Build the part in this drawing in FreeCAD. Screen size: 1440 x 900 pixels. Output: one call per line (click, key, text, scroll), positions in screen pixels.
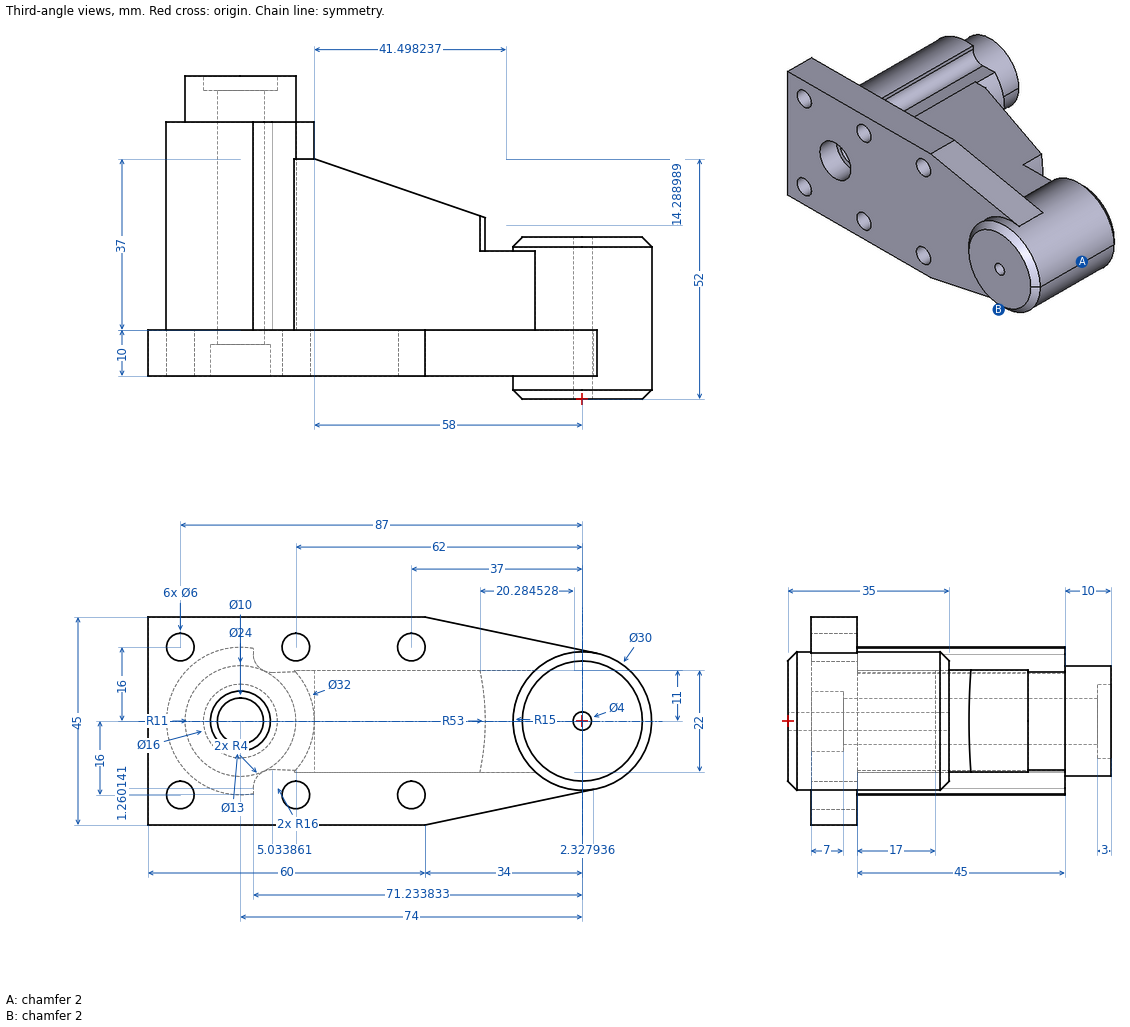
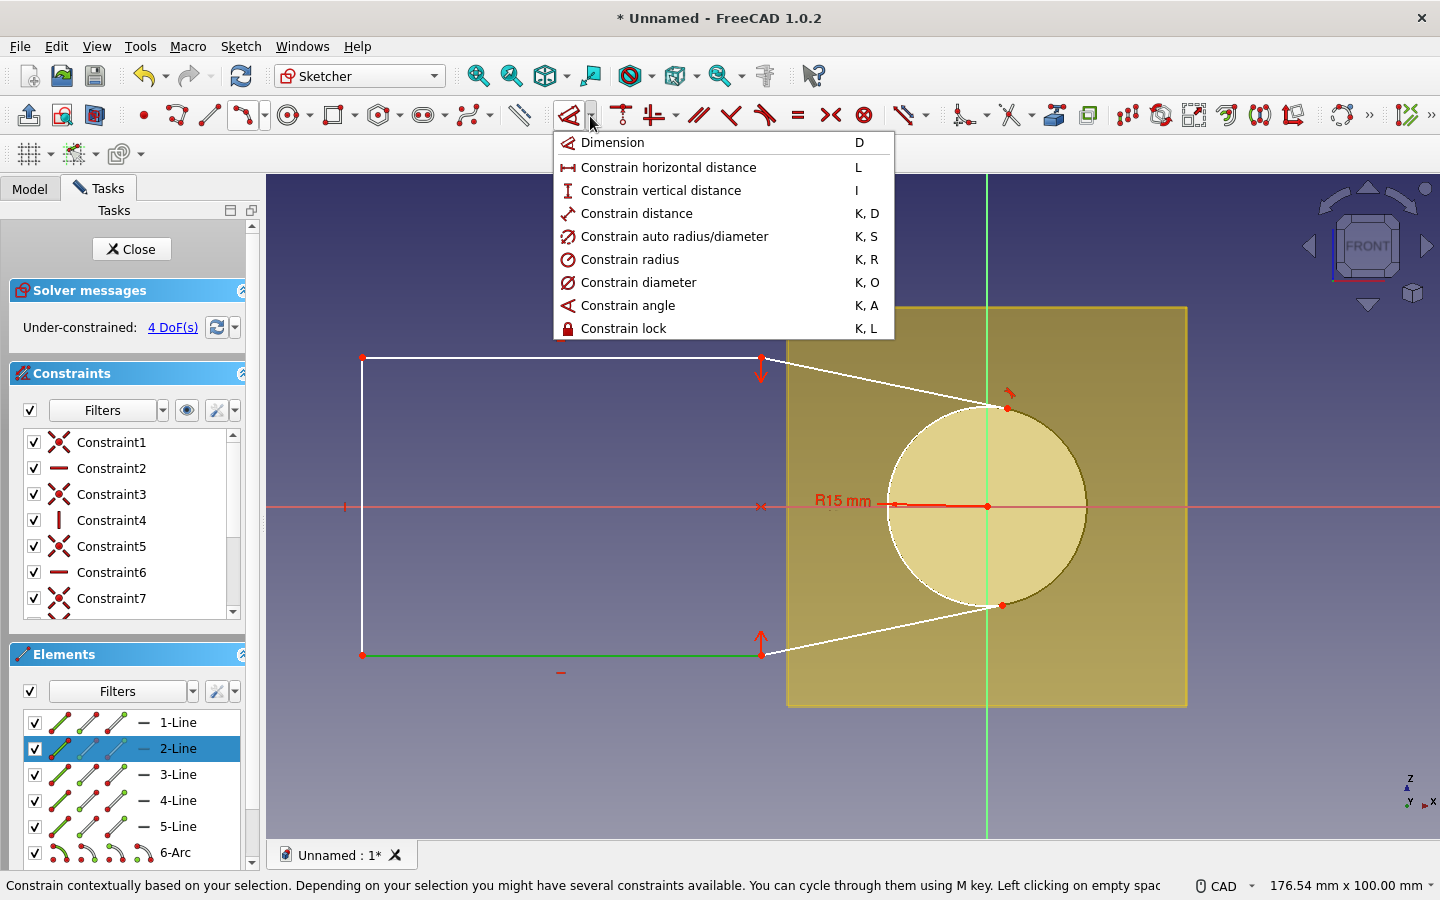
click(724, 168)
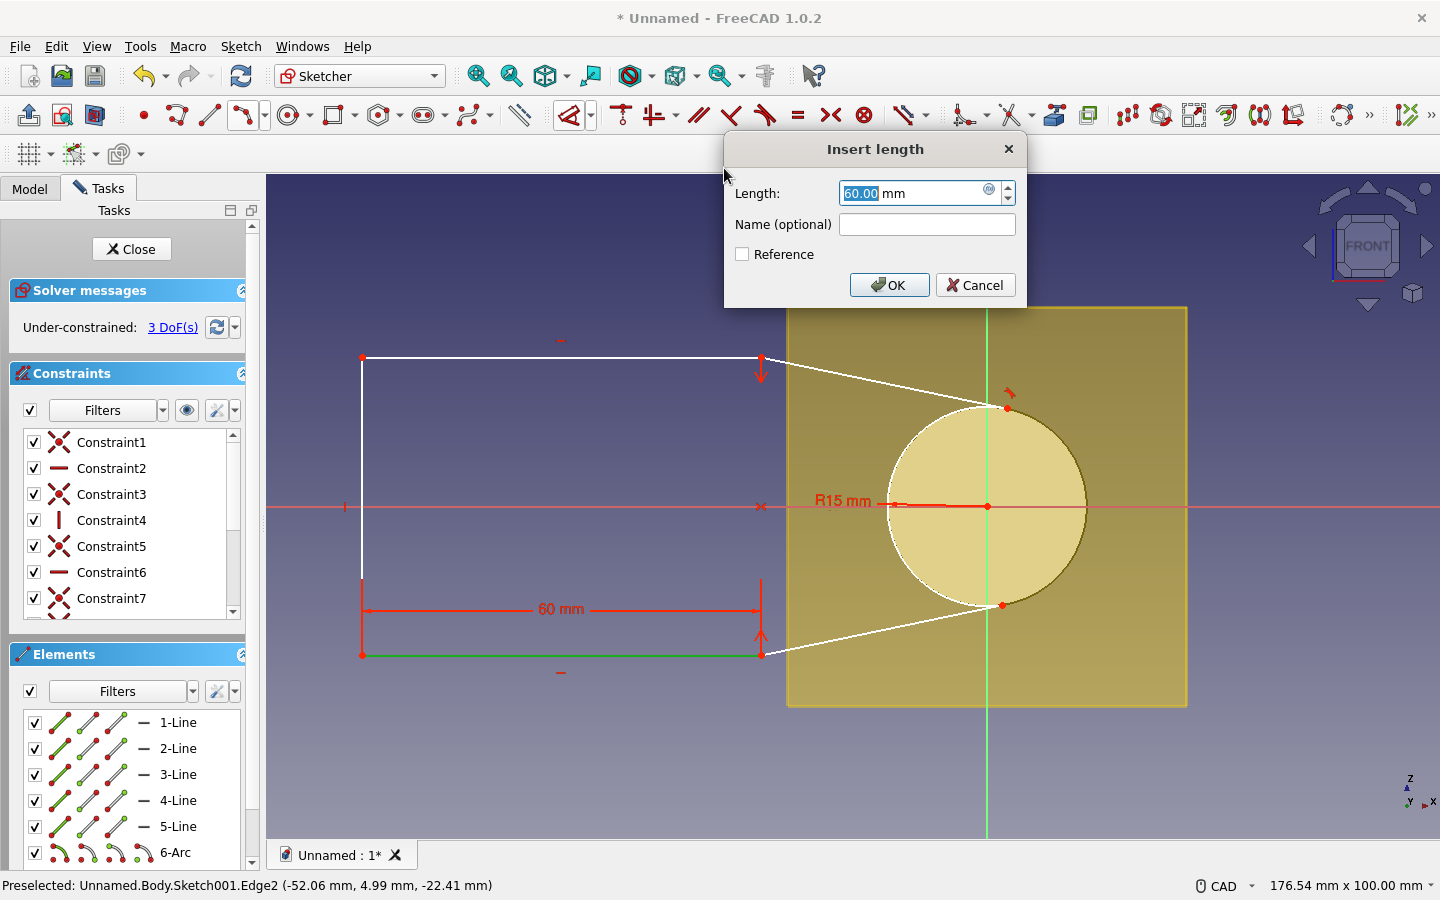
text(60)
key(Return)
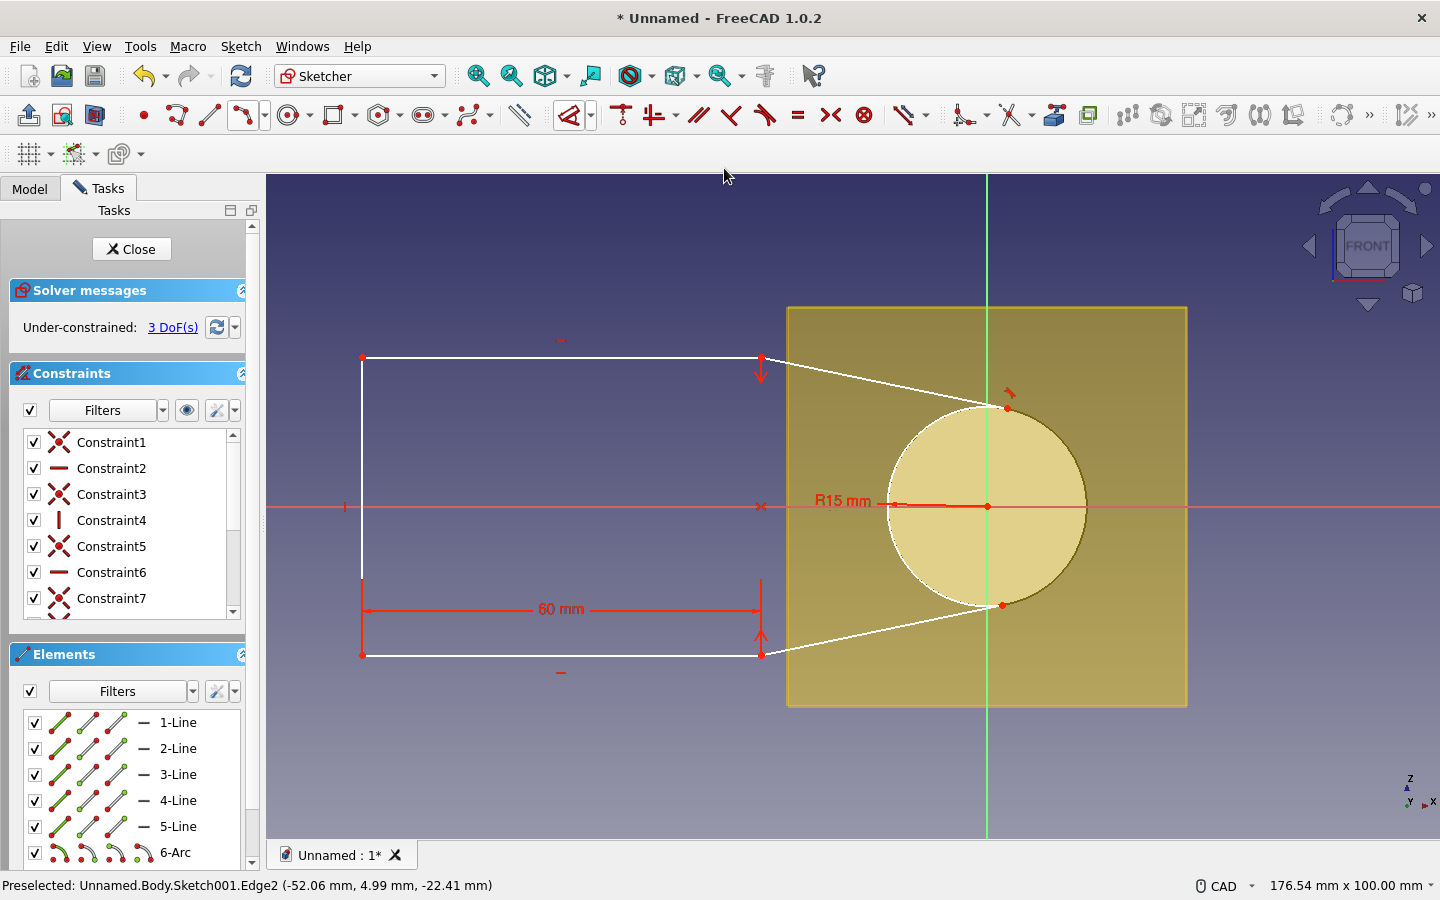
click(362, 566)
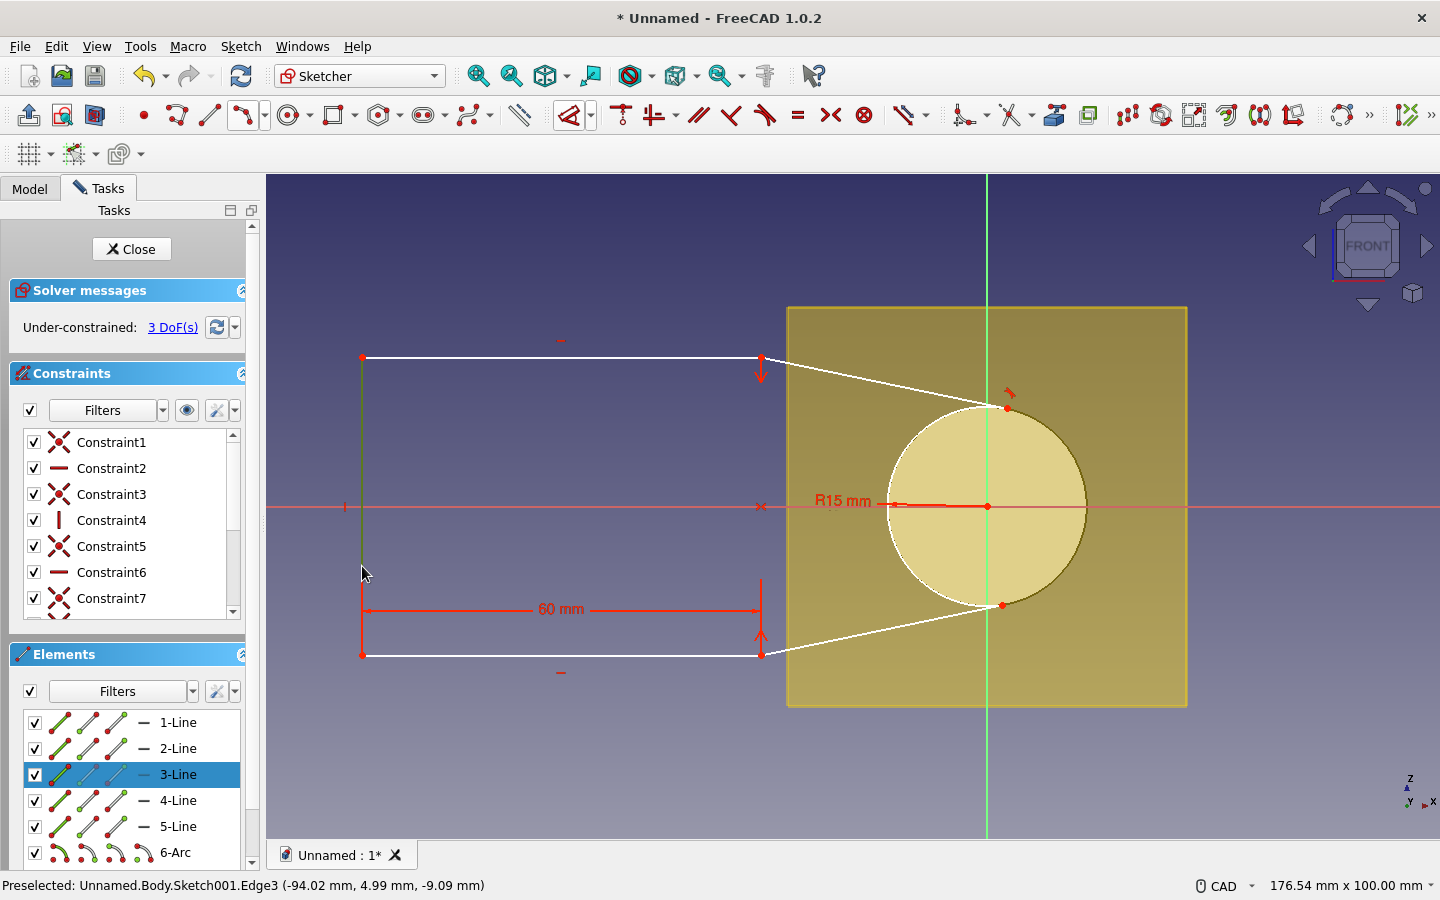
click(590, 116)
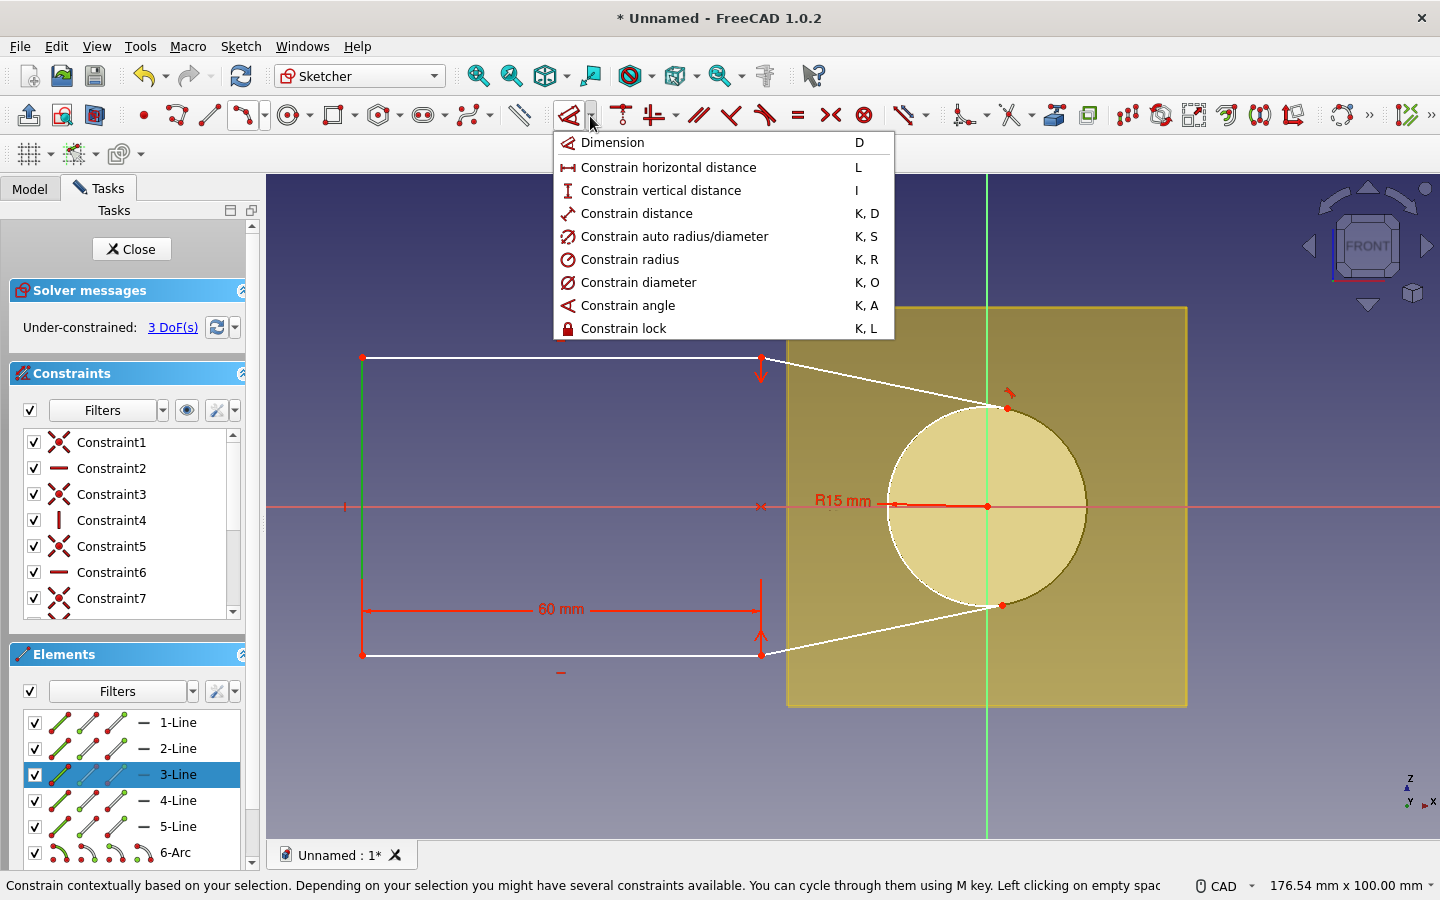
click(724, 190)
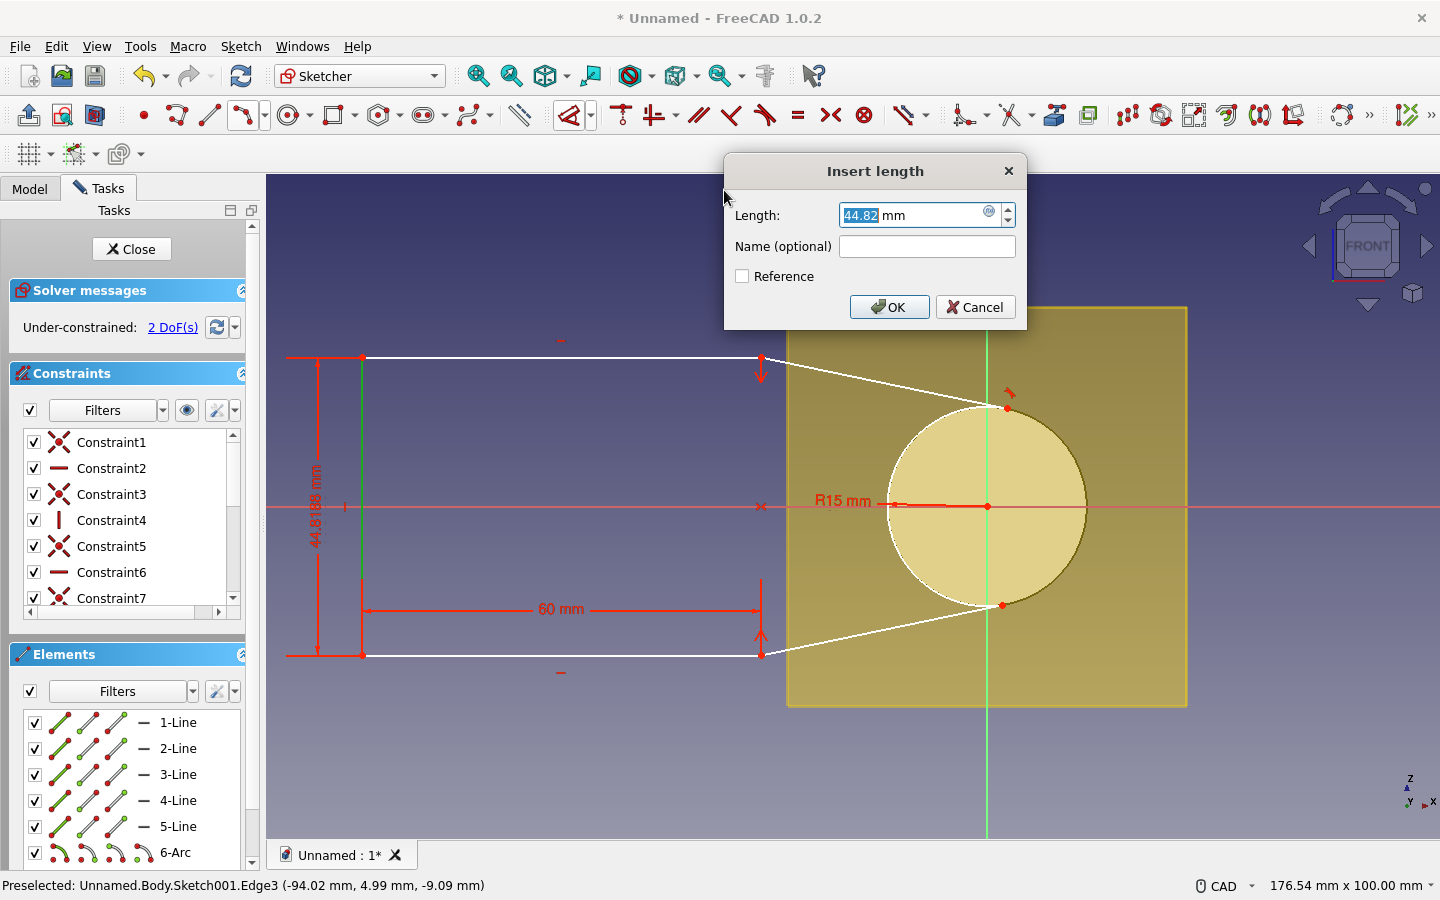
text(45)
key(Return)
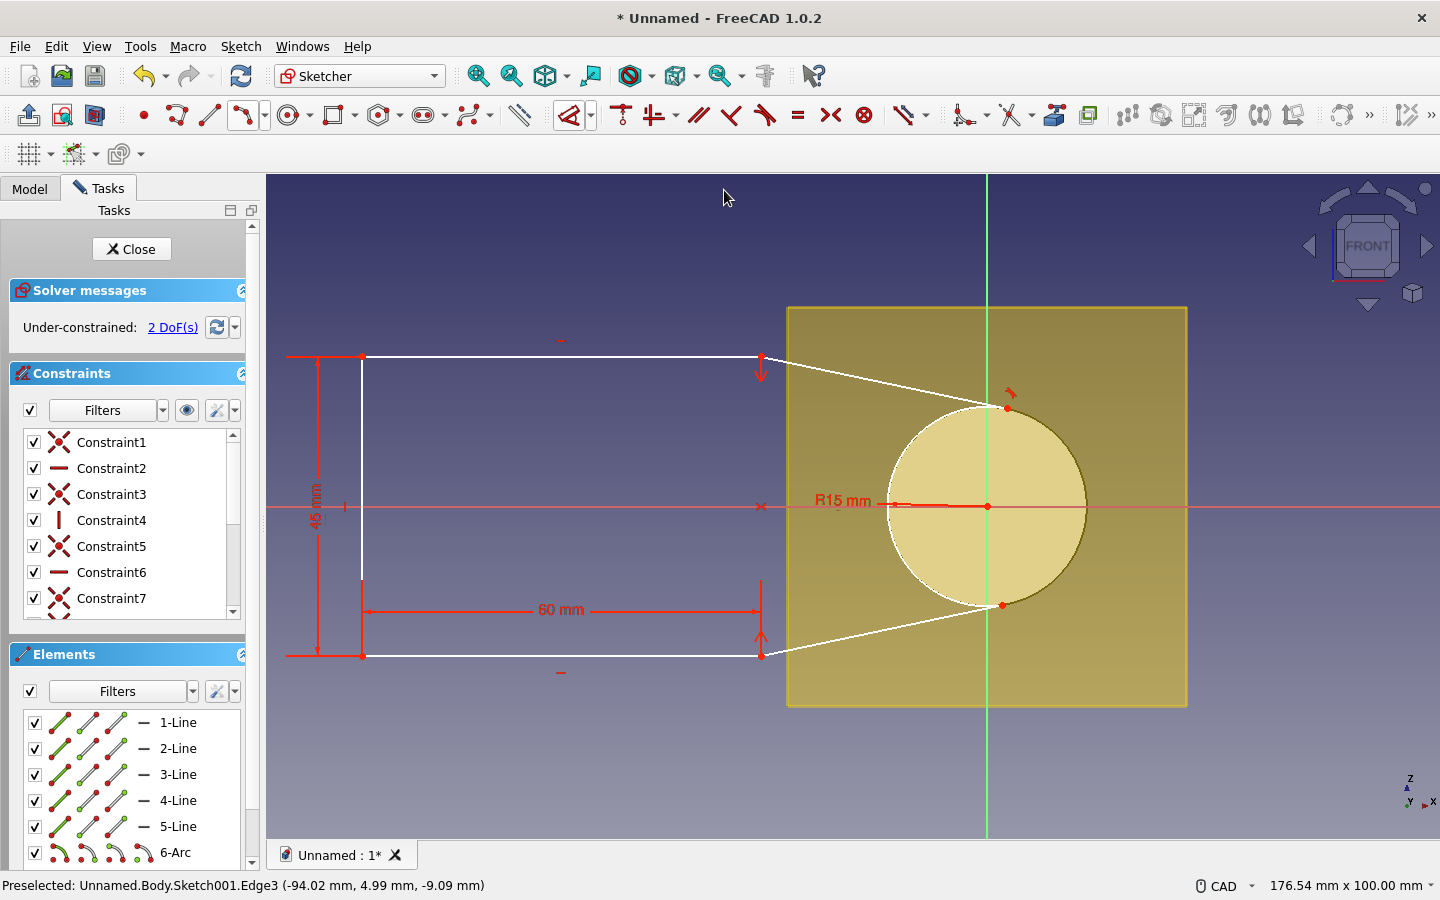
click(761, 656)